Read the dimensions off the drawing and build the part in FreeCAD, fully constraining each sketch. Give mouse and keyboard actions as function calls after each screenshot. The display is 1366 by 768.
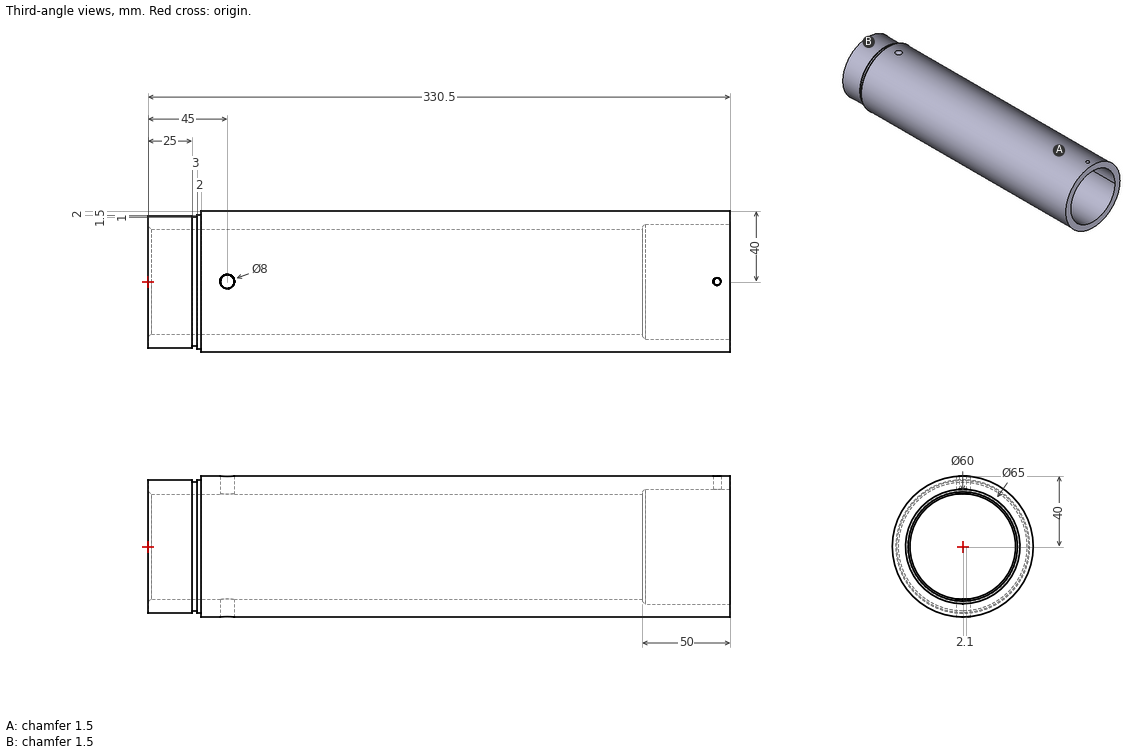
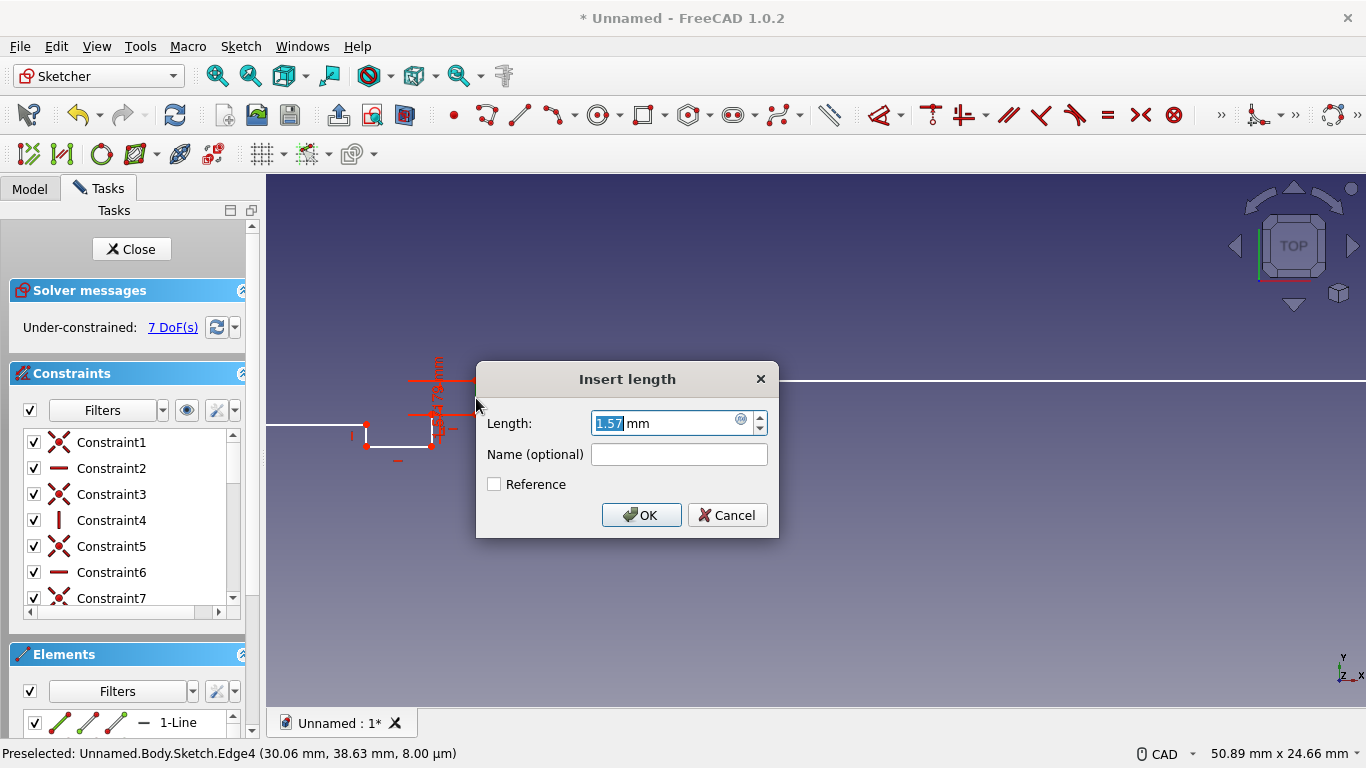
text(2)
key(Return)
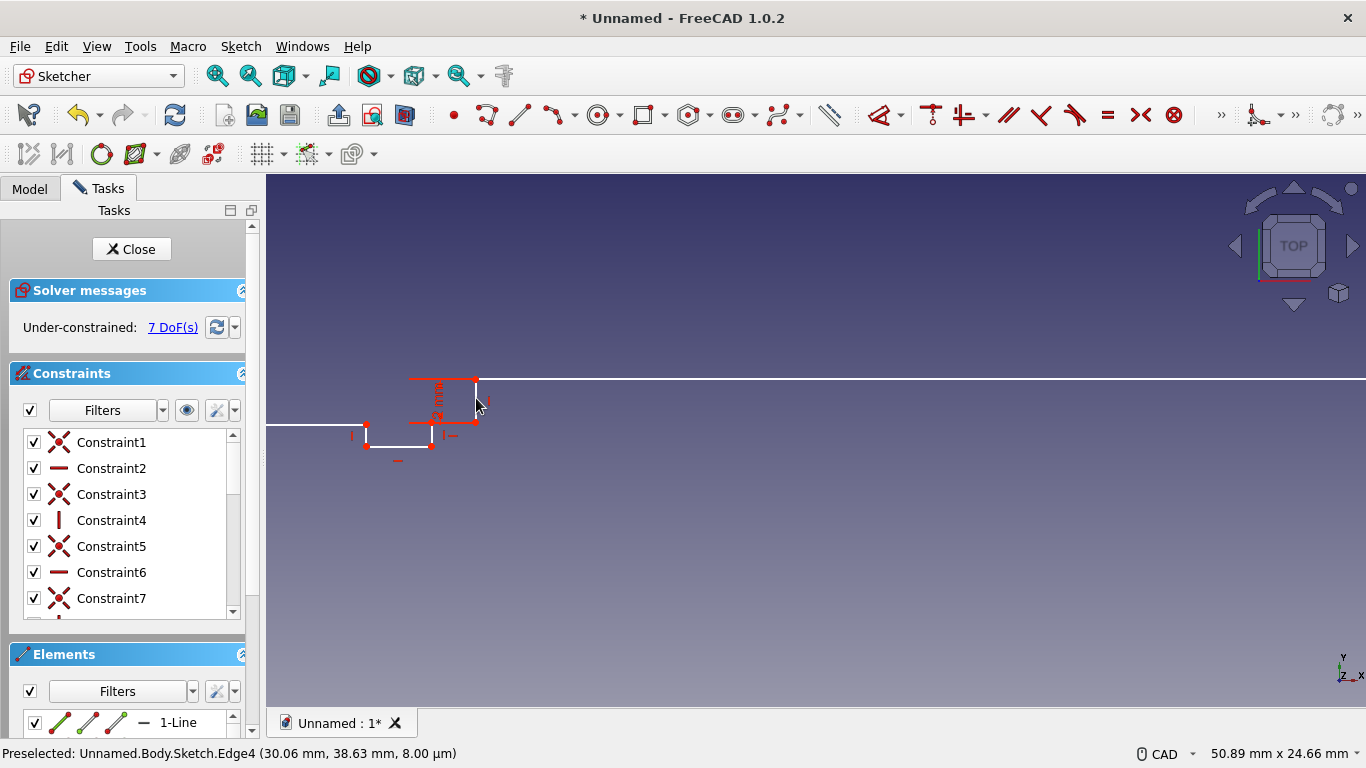
click(463, 423)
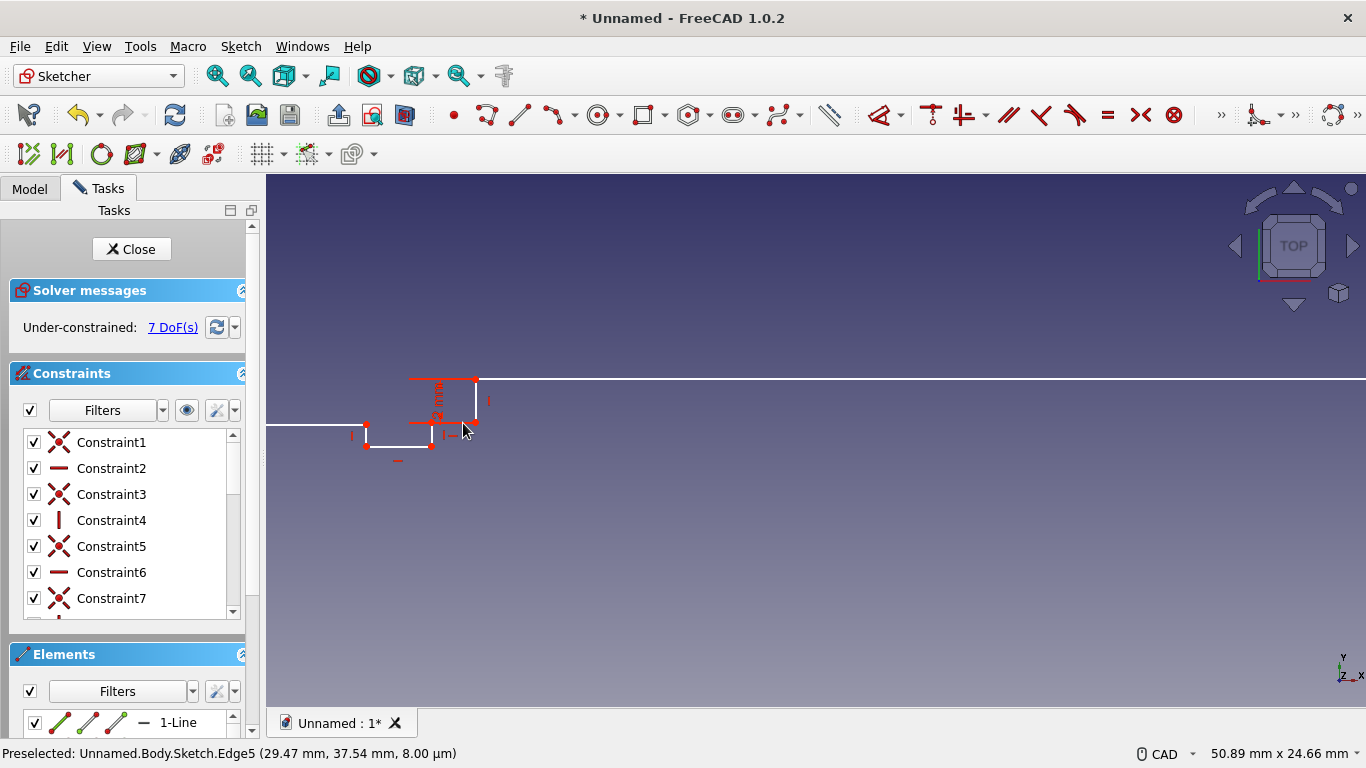
key(l)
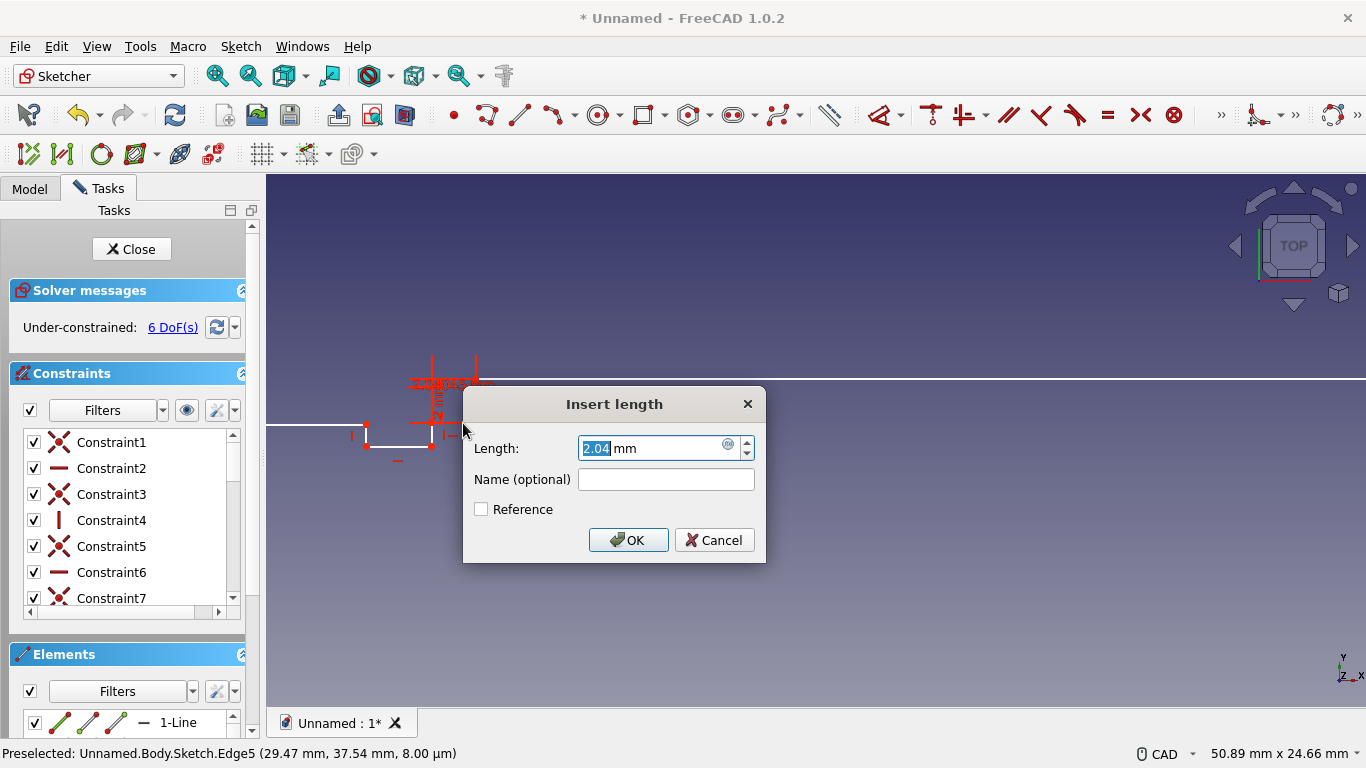
text(2)
key(Return)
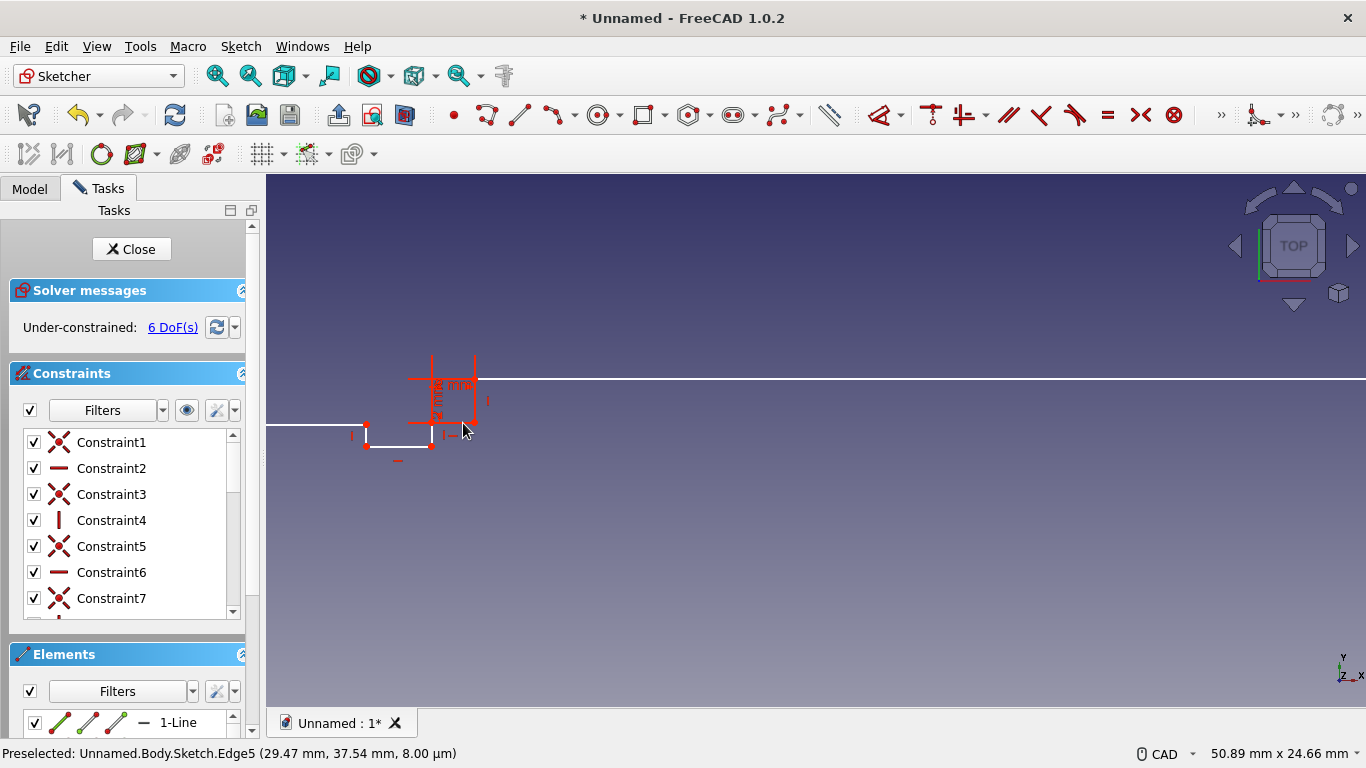
click(412, 447)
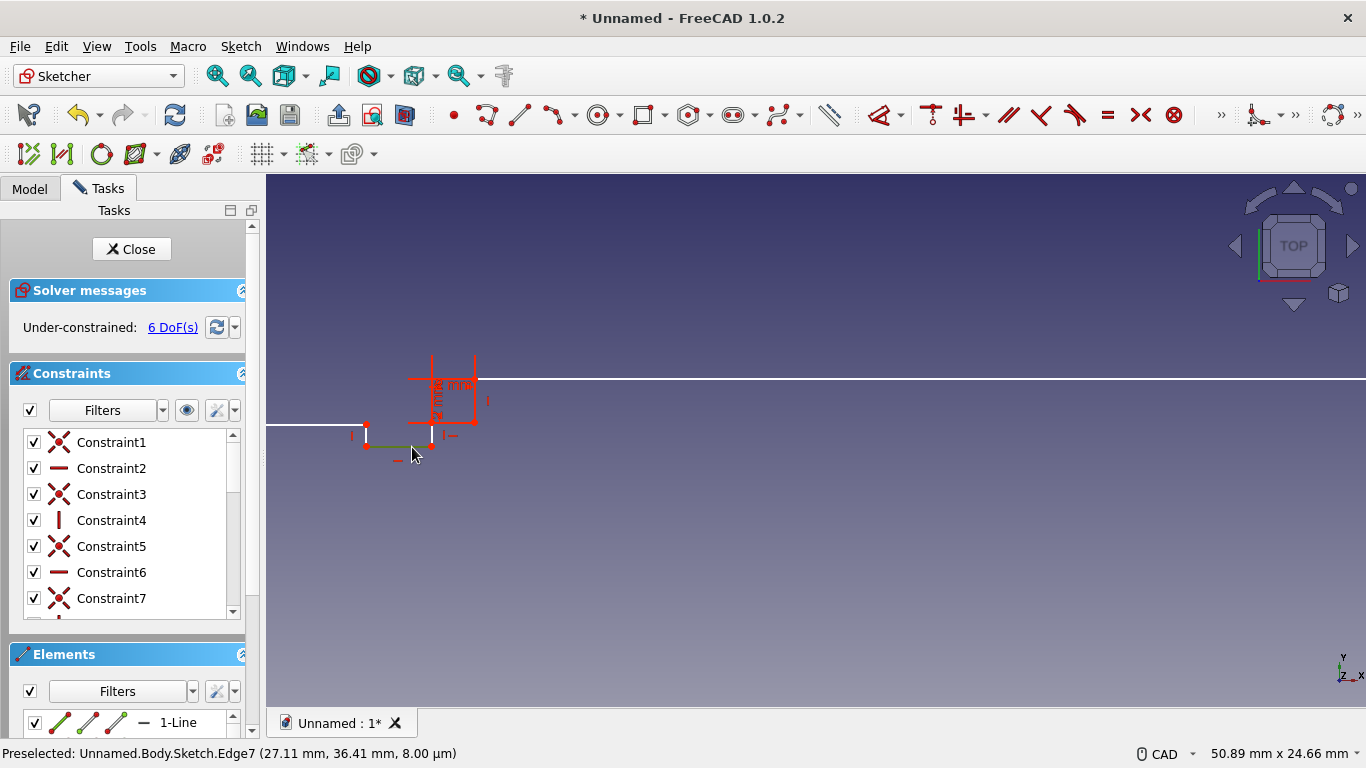
click(900, 116)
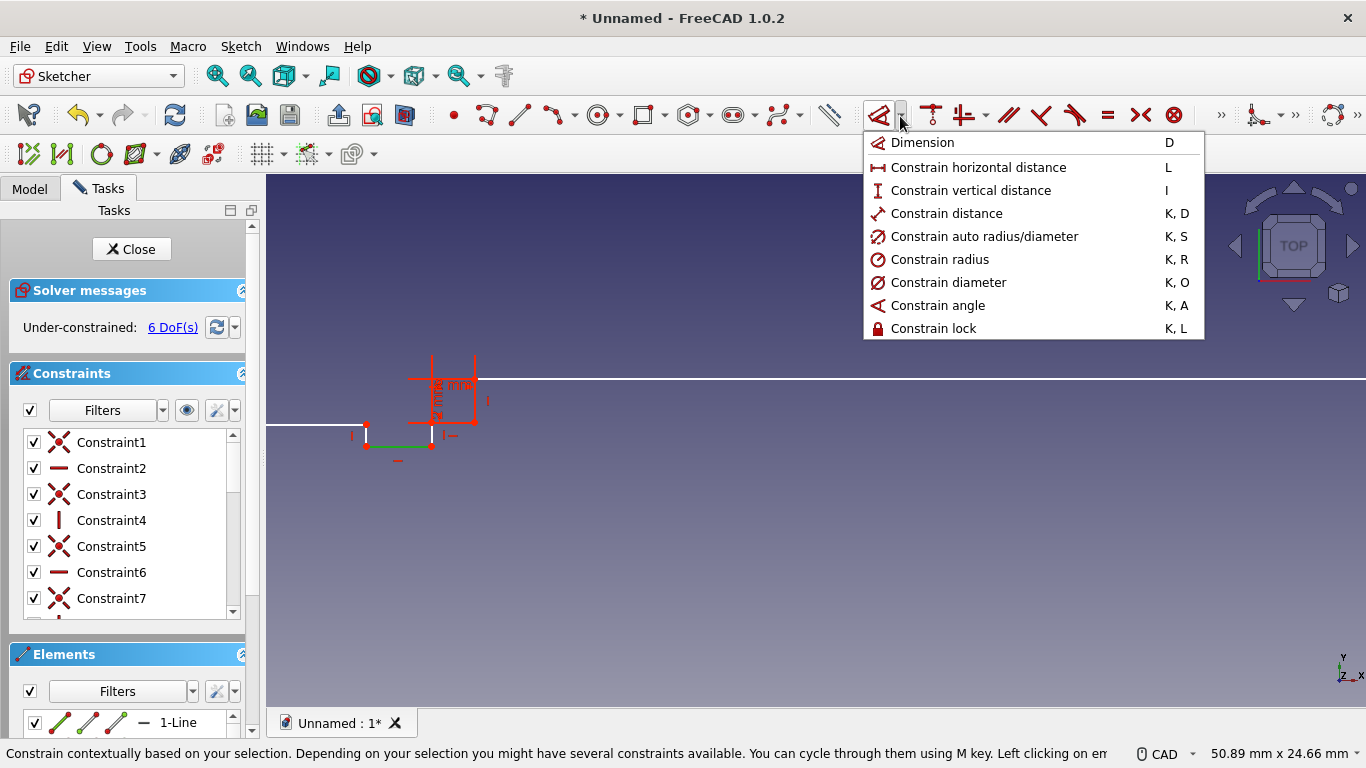
click(1034, 168)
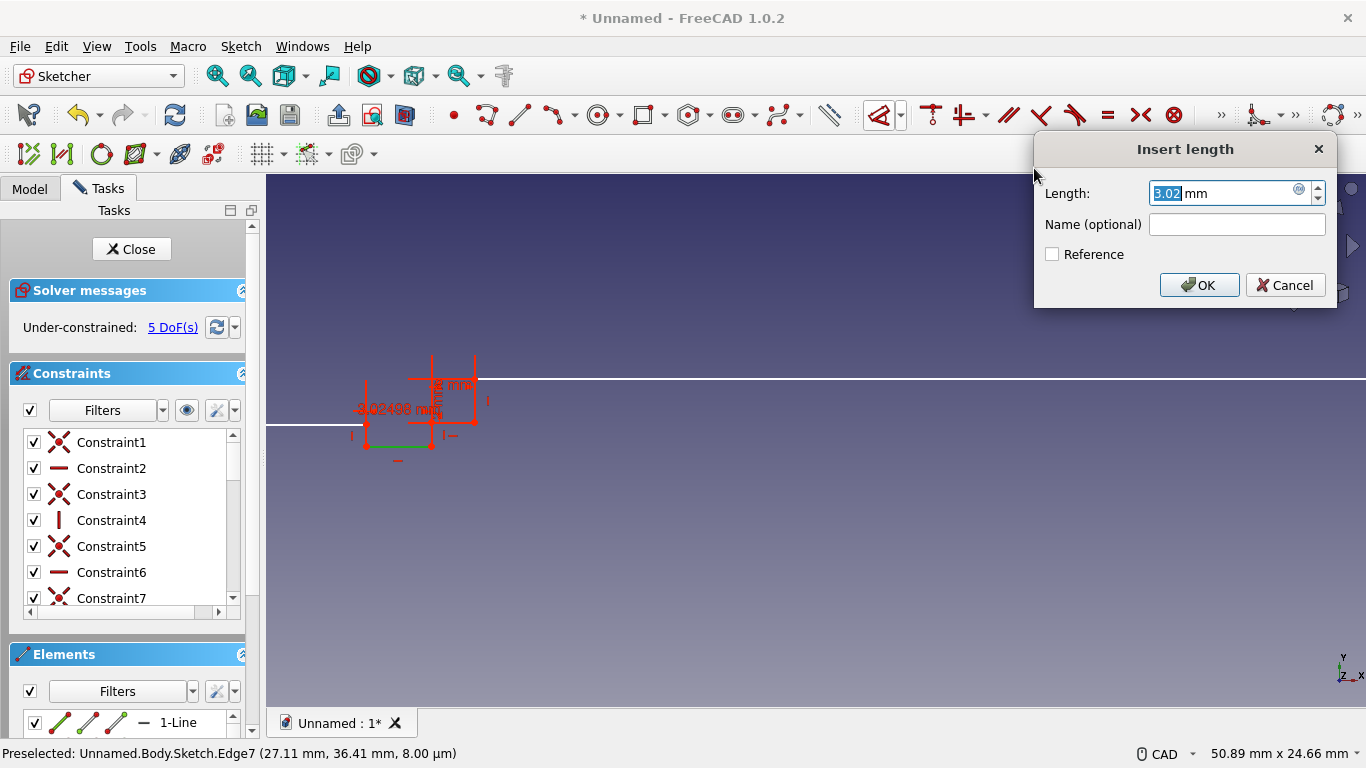
text(3)
key(Return)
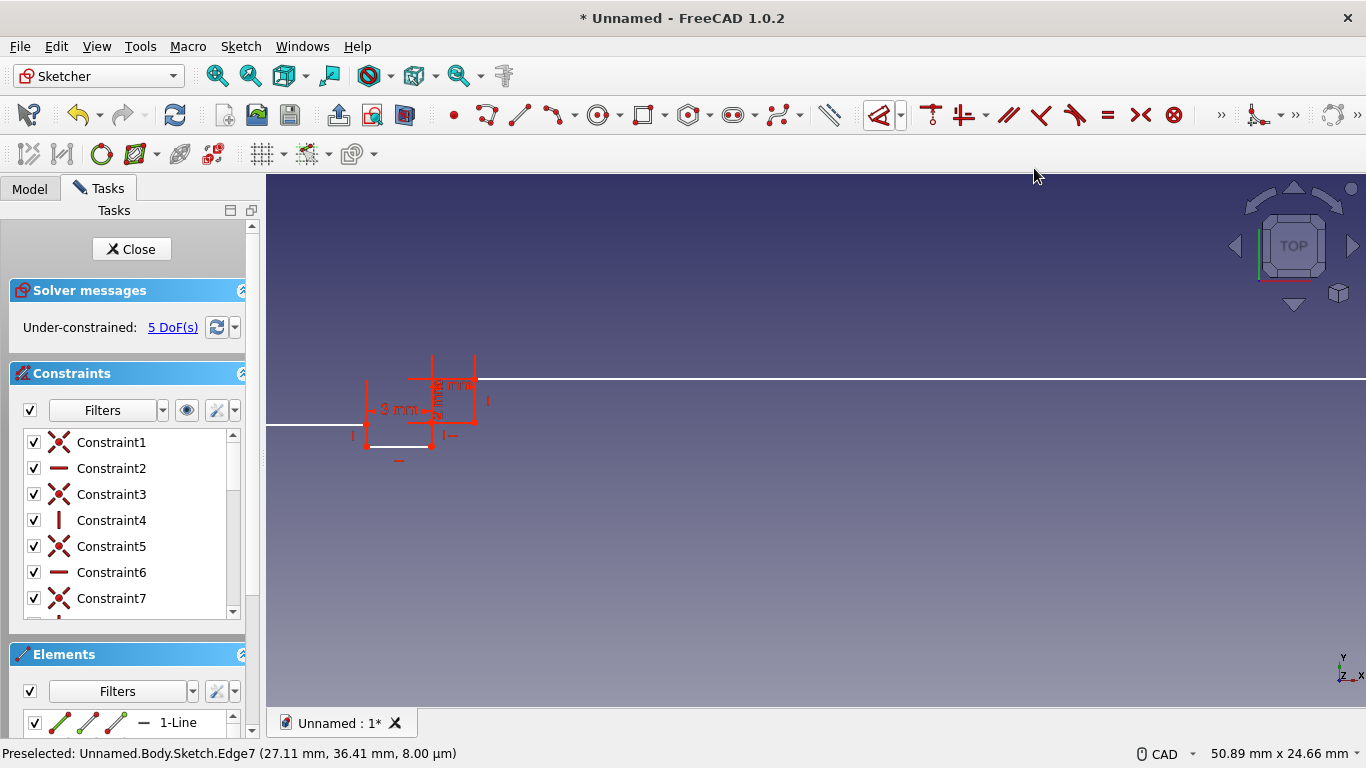
scroll(367, 436, up, 4)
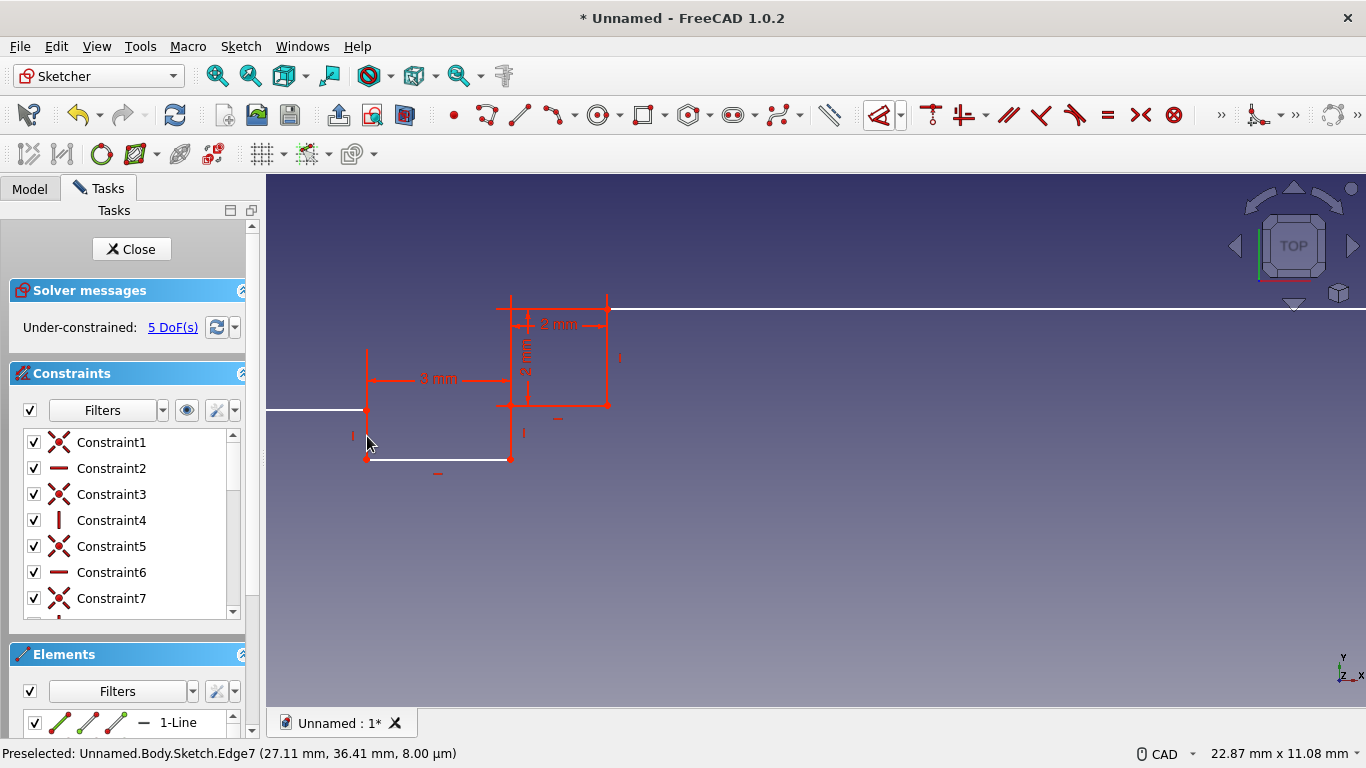
click(367, 435)